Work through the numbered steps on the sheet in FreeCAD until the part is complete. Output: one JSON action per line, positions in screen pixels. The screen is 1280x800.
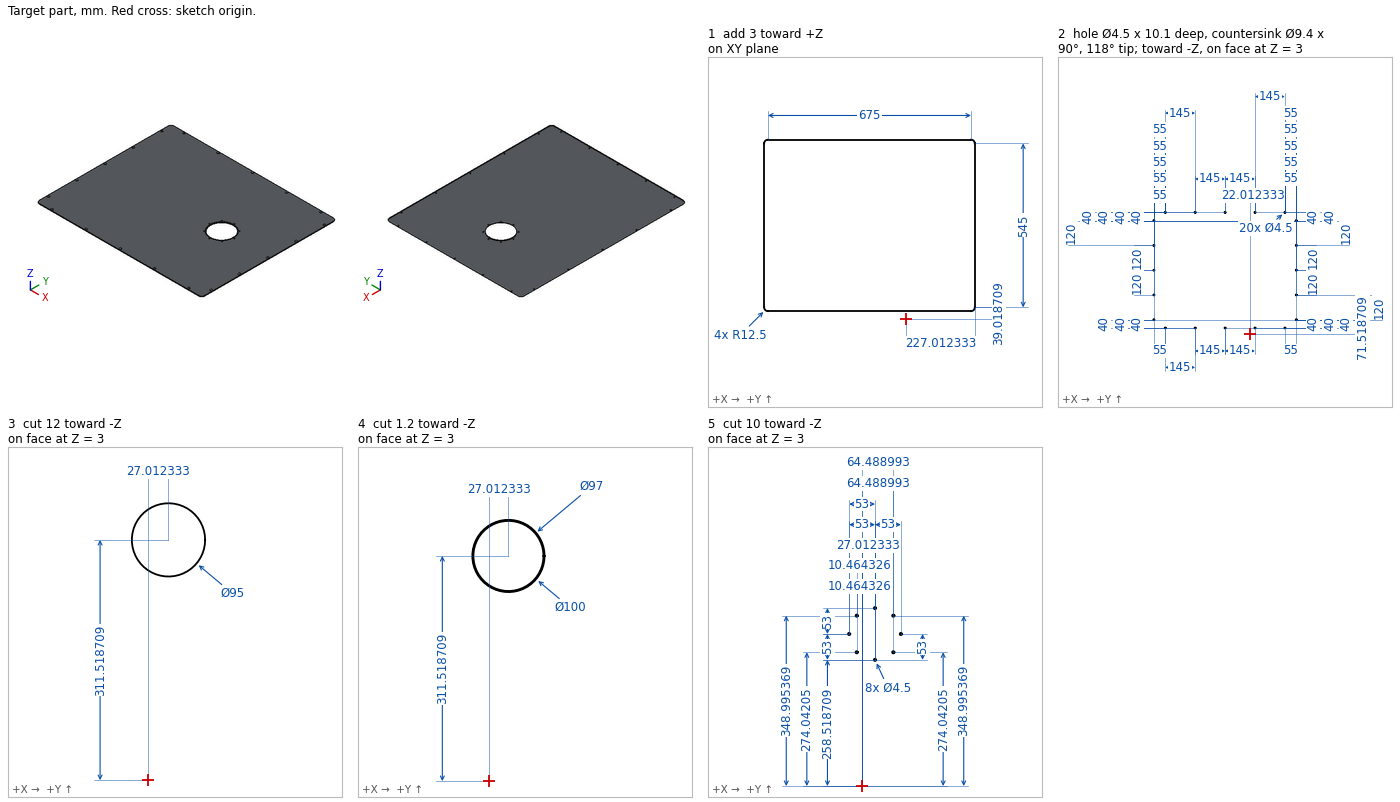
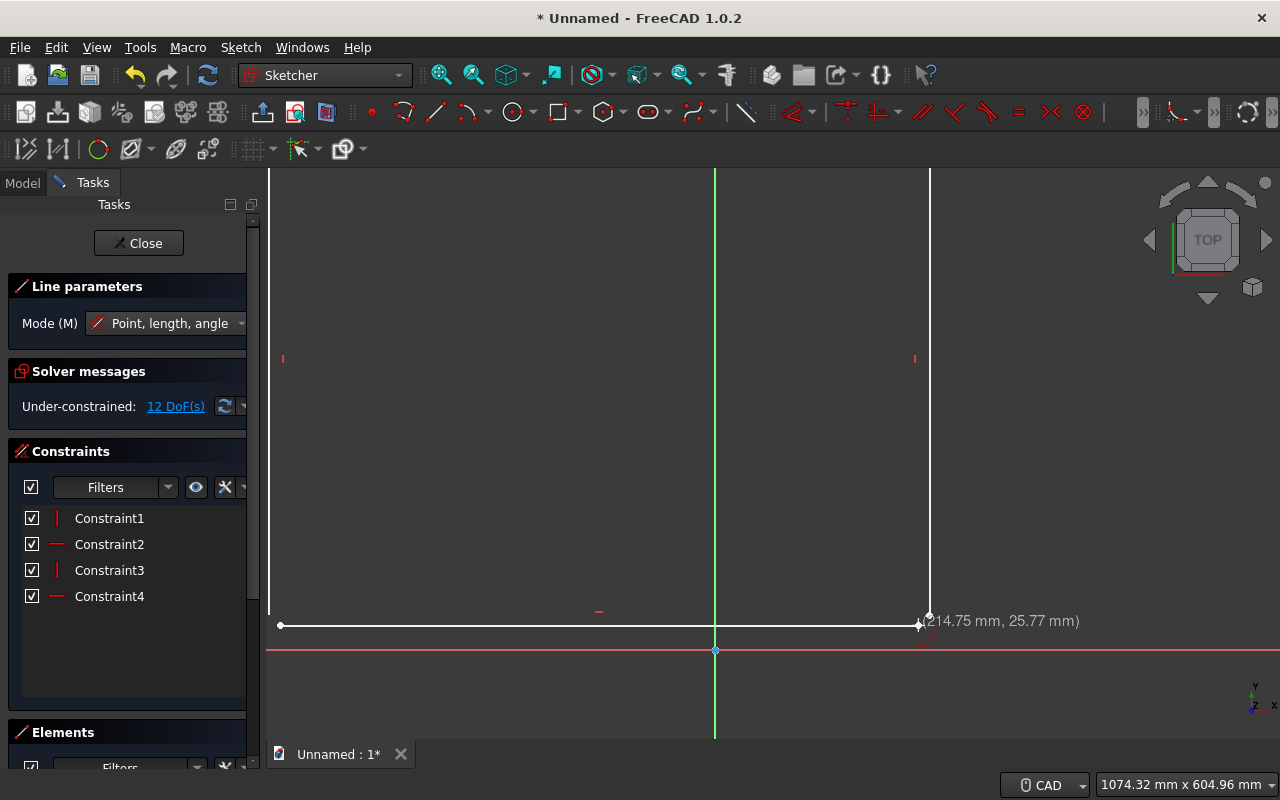
{"action": "key", "text": "g 3 a"}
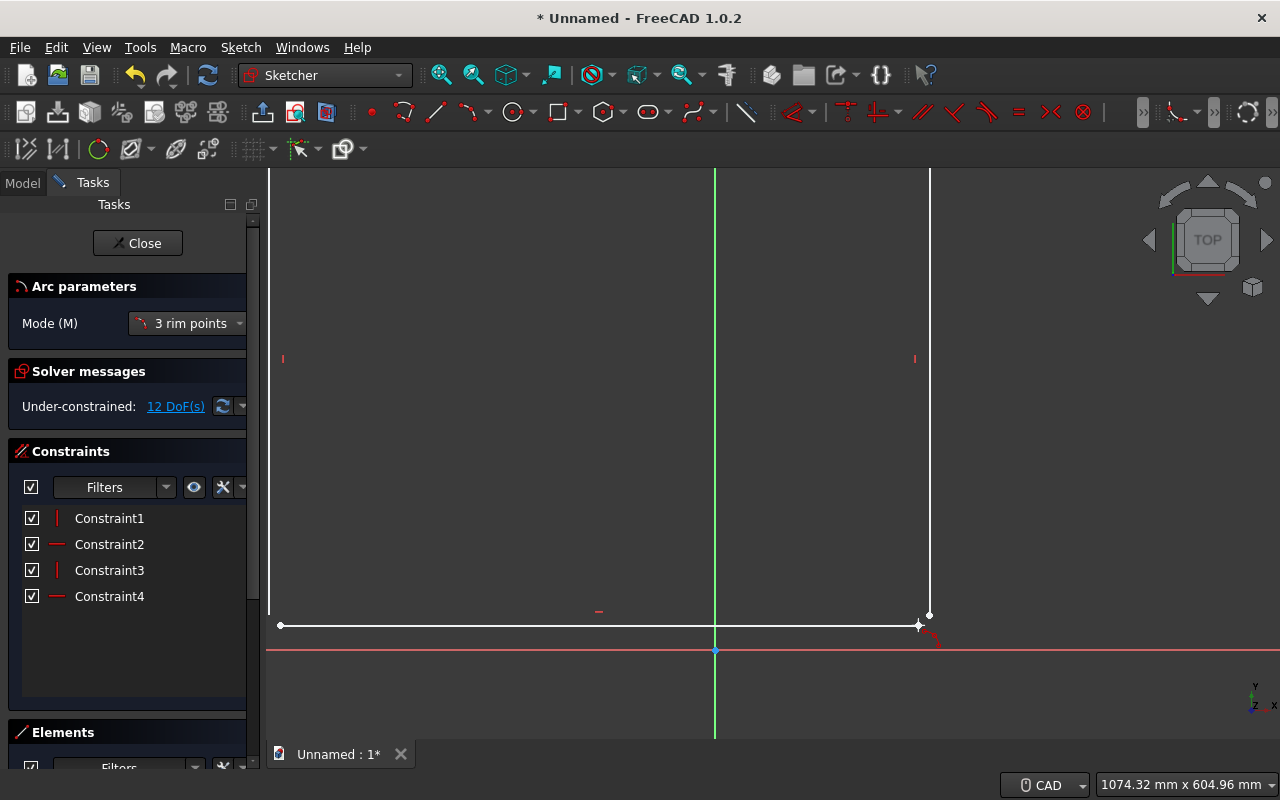
{"action": "scroll", "coordinate": [919, 626], "scroll_direction": "down", "scroll_amount": 2}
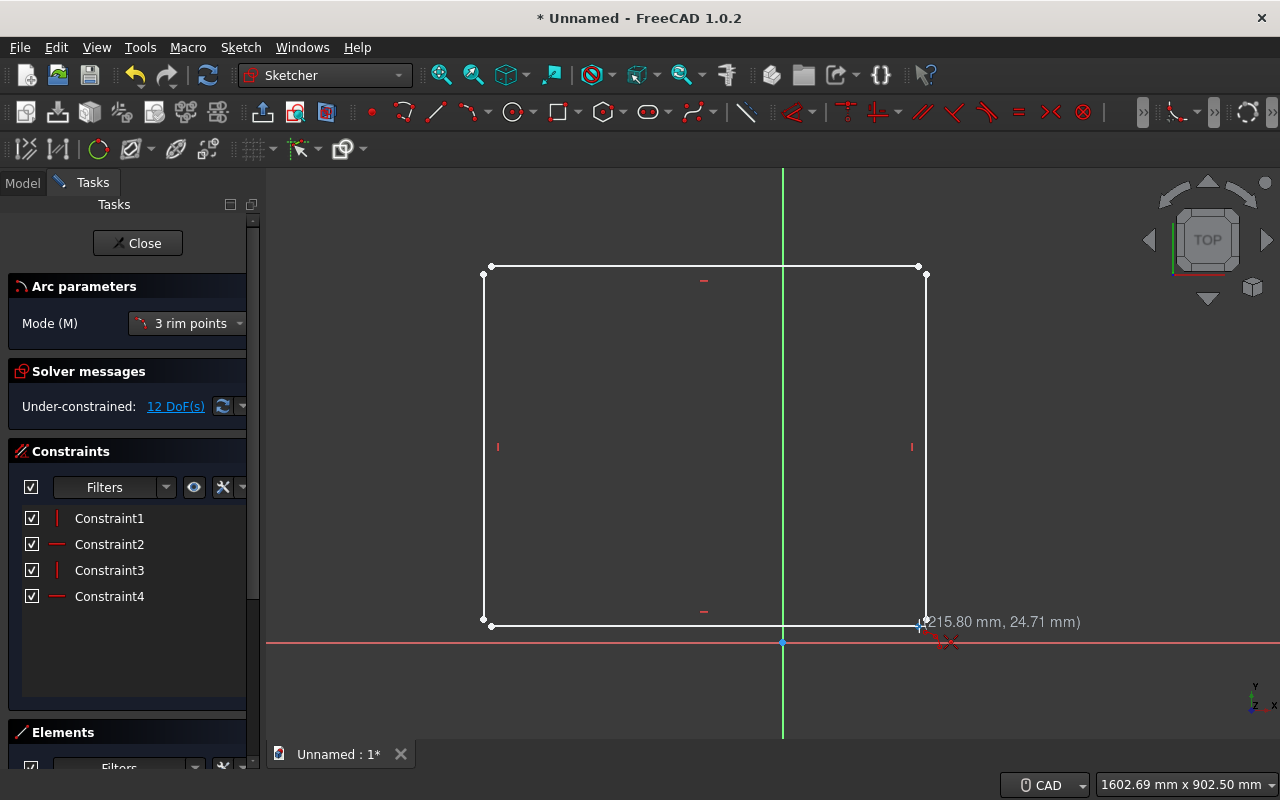
{"action": "scroll", "coordinate": [926, 273], "scroll_direction": "up", "scroll_amount": 2}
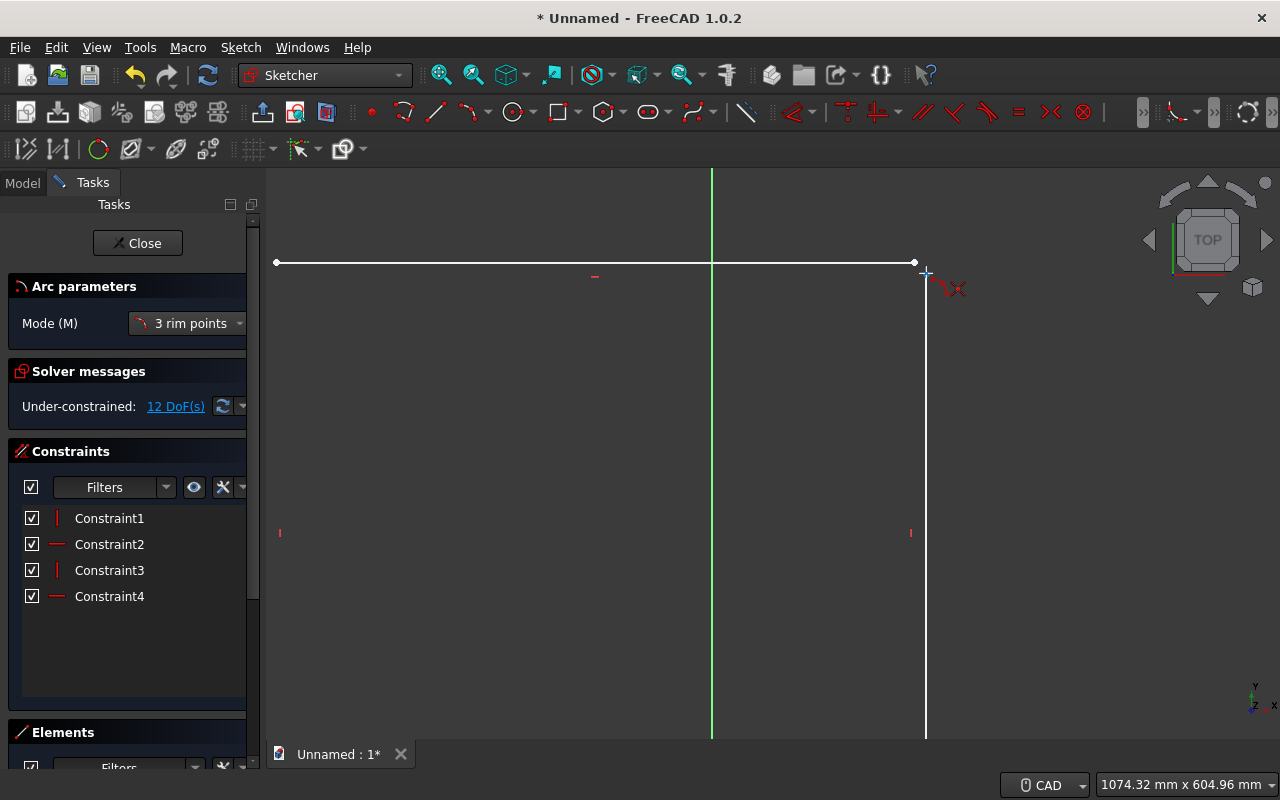
{"action": "left_click", "coordinate": [926, 275]}
{"action": "left_click", "coordinate": [915, 263]}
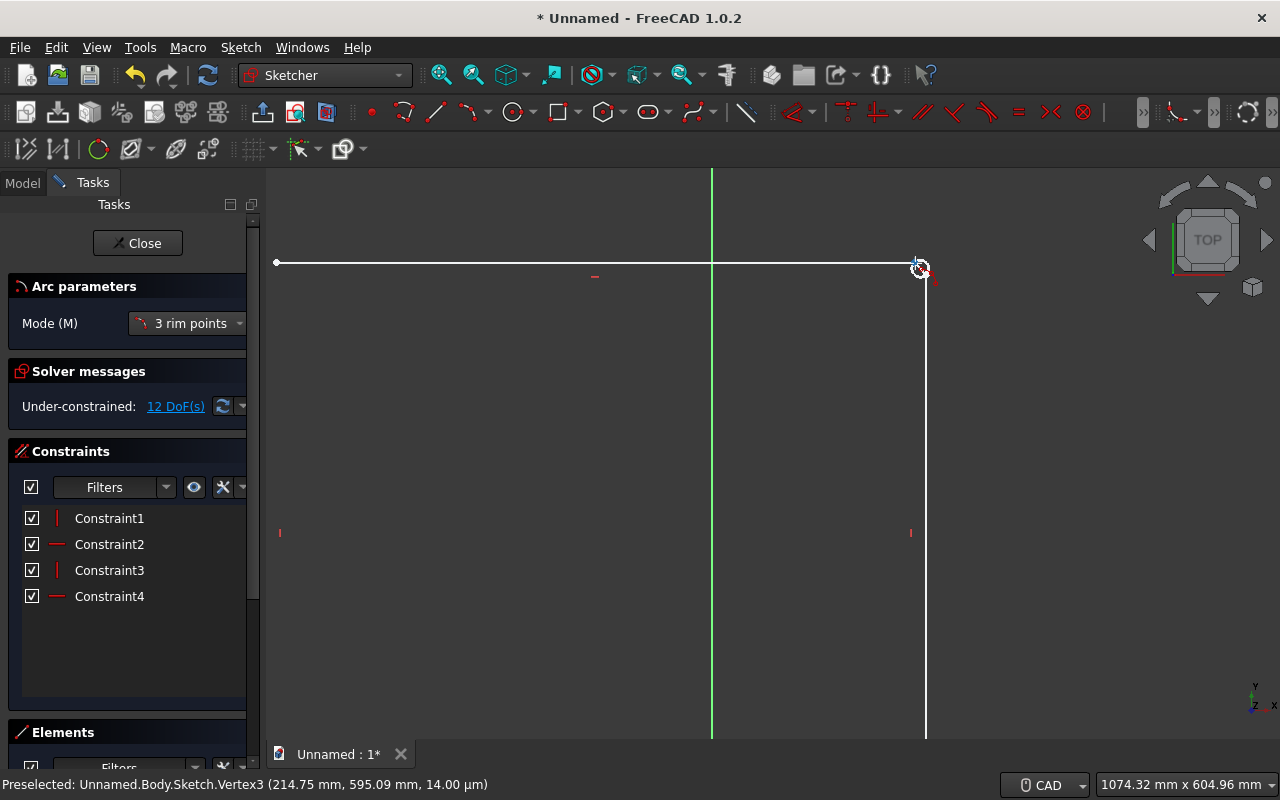
{"action": "scroll", "coordinate": [923, 265], "scroll_direction": "up", "scroll_amount": 8}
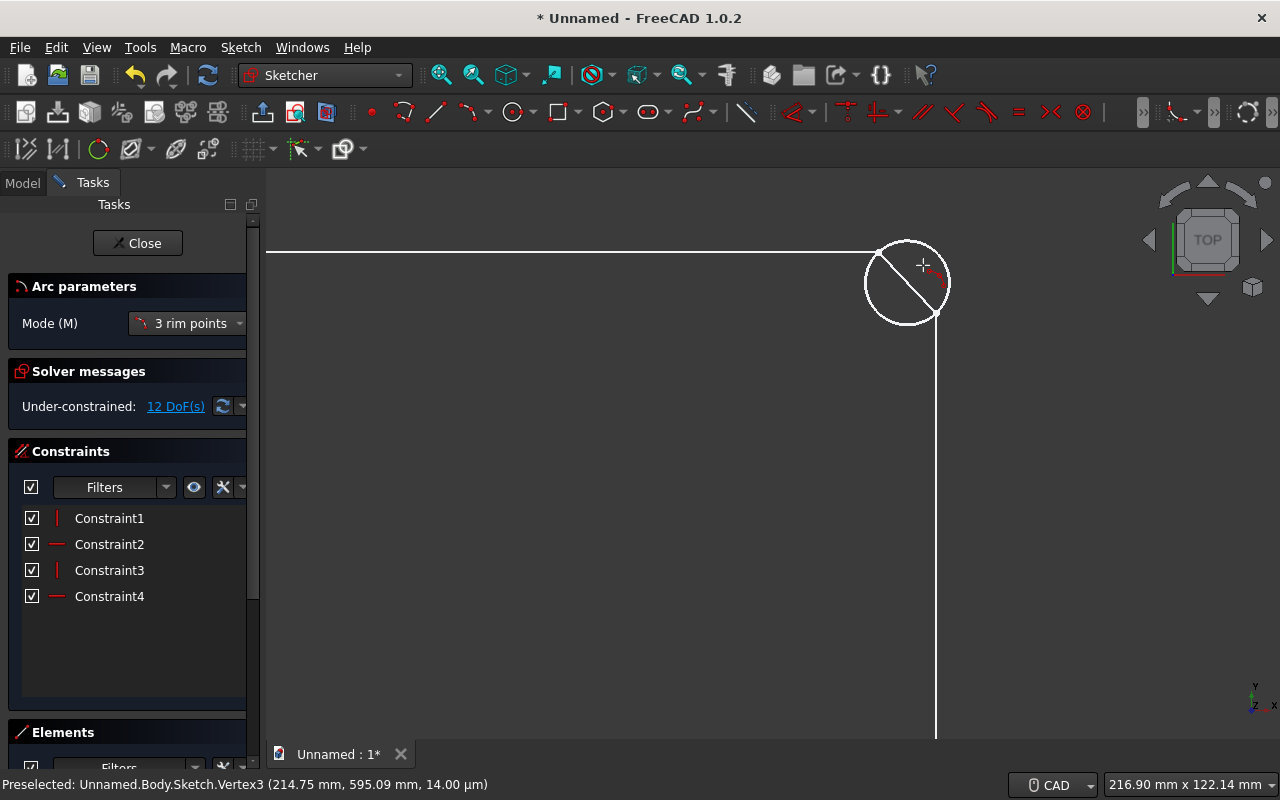
{"action": "left_click", "coordinate": [919, 263]}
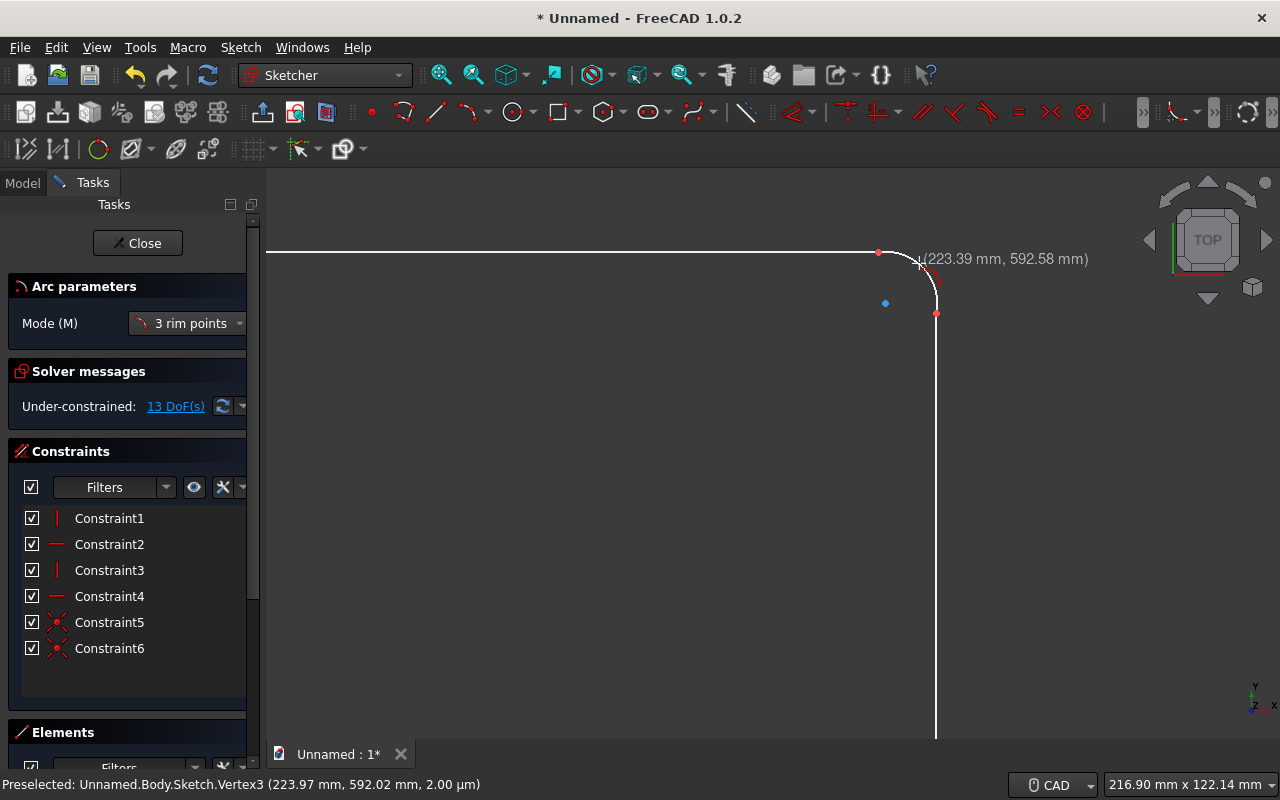
{"action": "scroll", "coordinate": [924, 268], "scroll_direction": "down", "scroll_amount": 10}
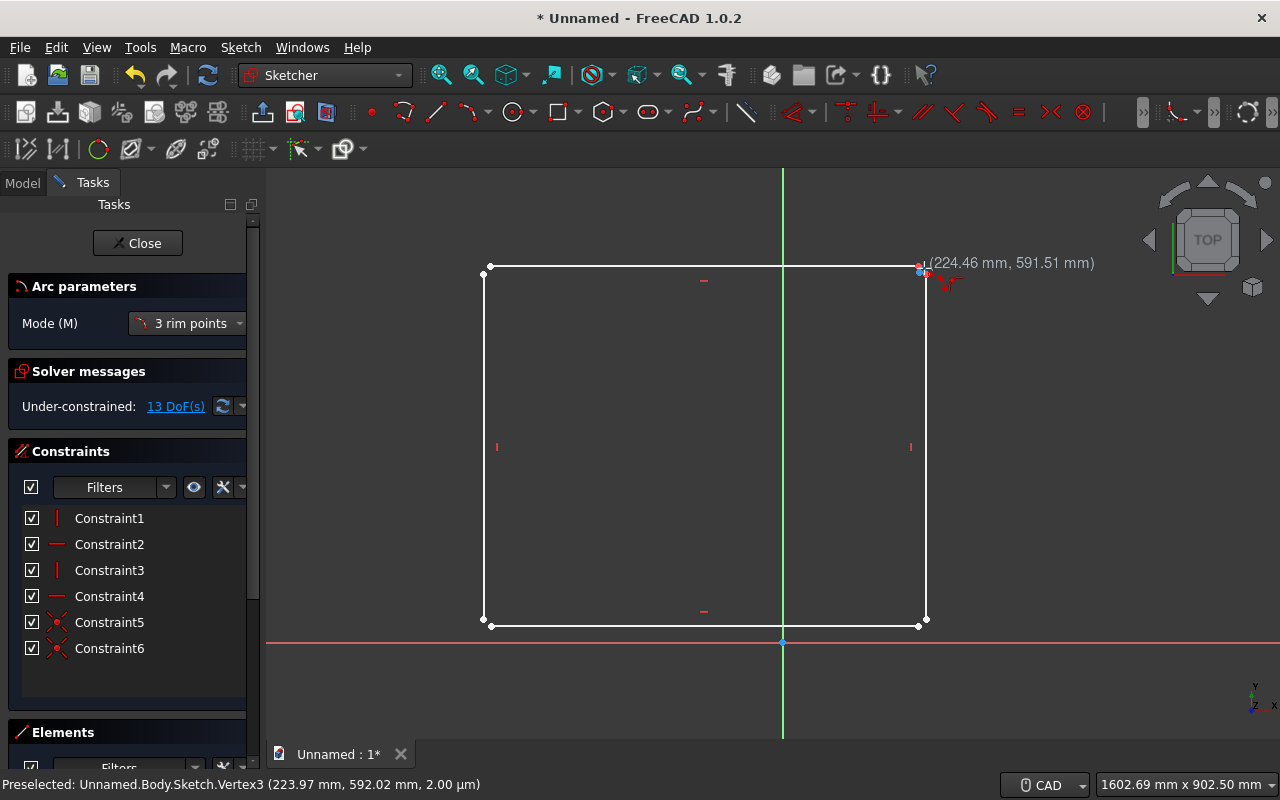
{"action": "scroll", "coordinate": [491, 265], "scroll_direction": "up", "scroll_amount": 2}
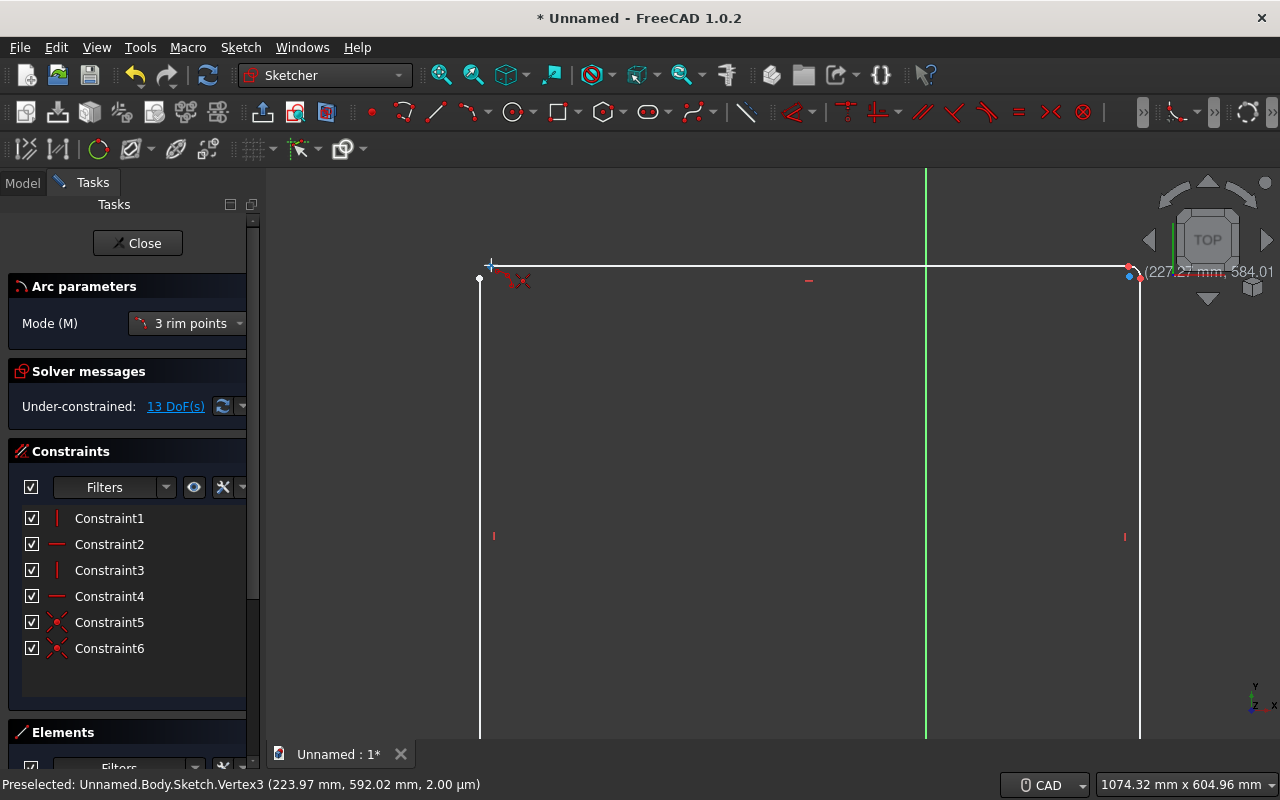
{"action": "left_click", "coordinate": [491, 266]}
{"action": "left_click", "coordinate": [480, 278]}